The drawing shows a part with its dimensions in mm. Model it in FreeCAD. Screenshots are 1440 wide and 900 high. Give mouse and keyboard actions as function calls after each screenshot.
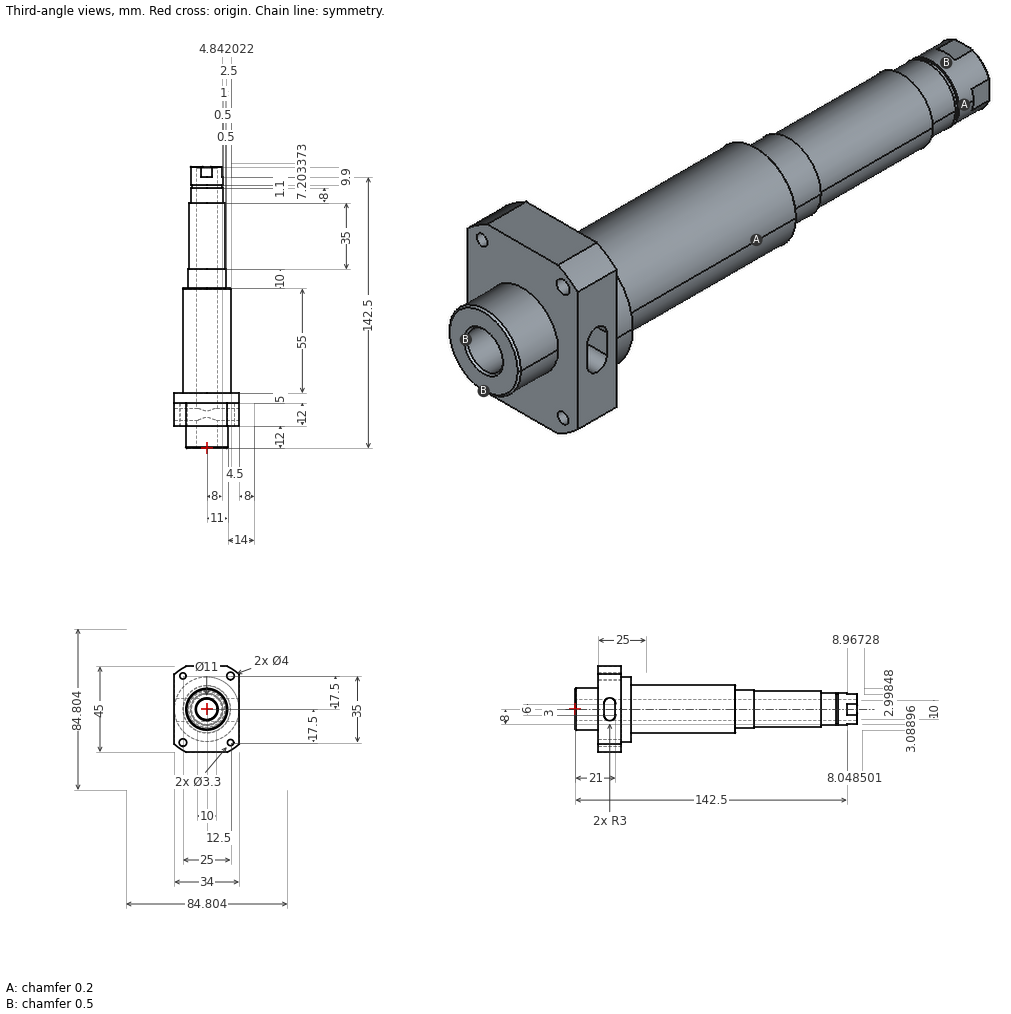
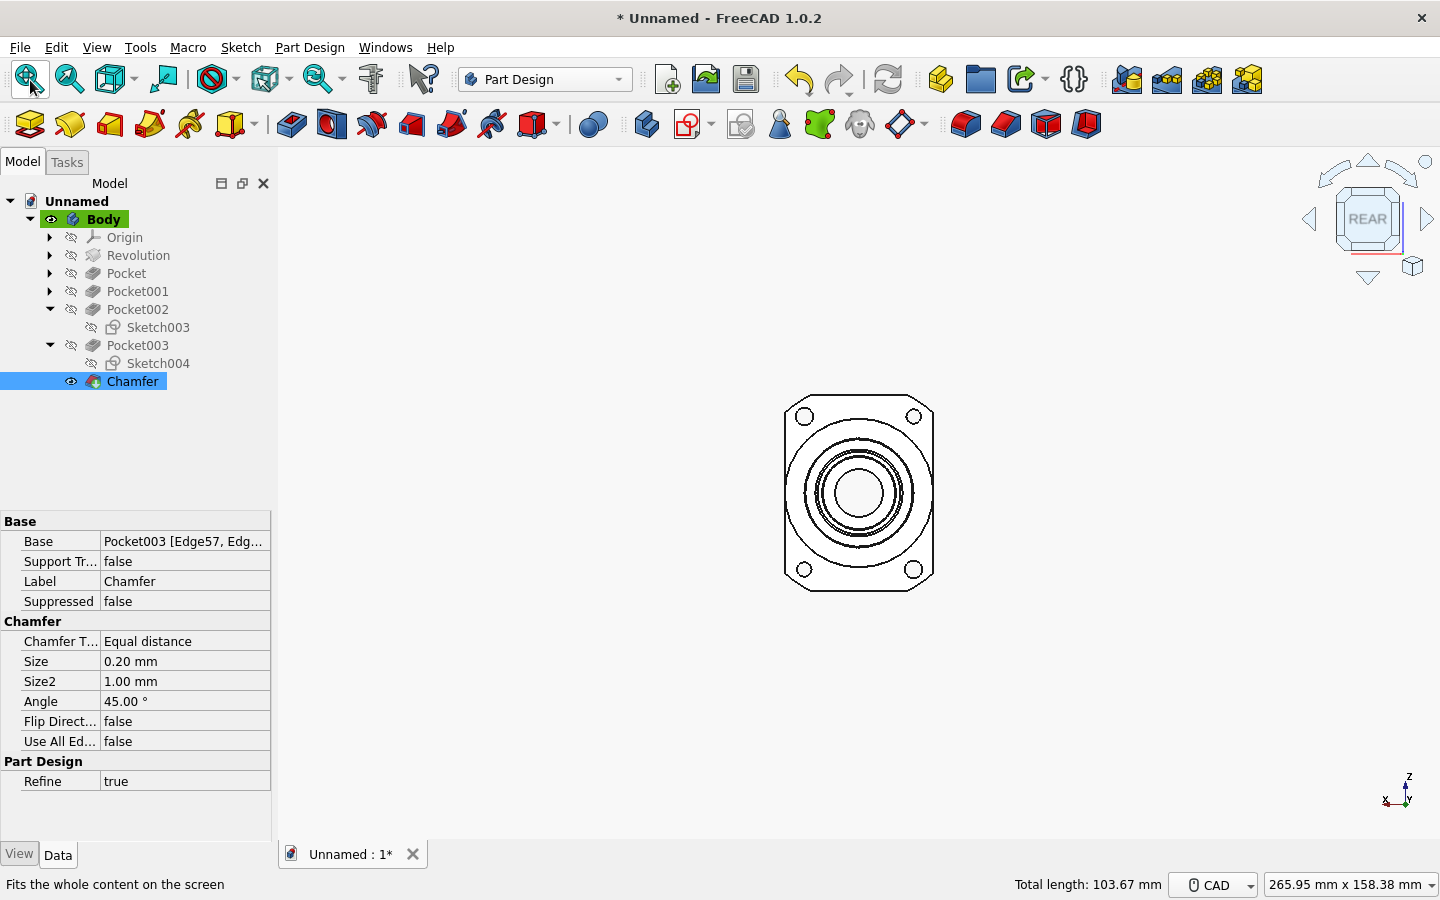
click(883, 492, ctrl)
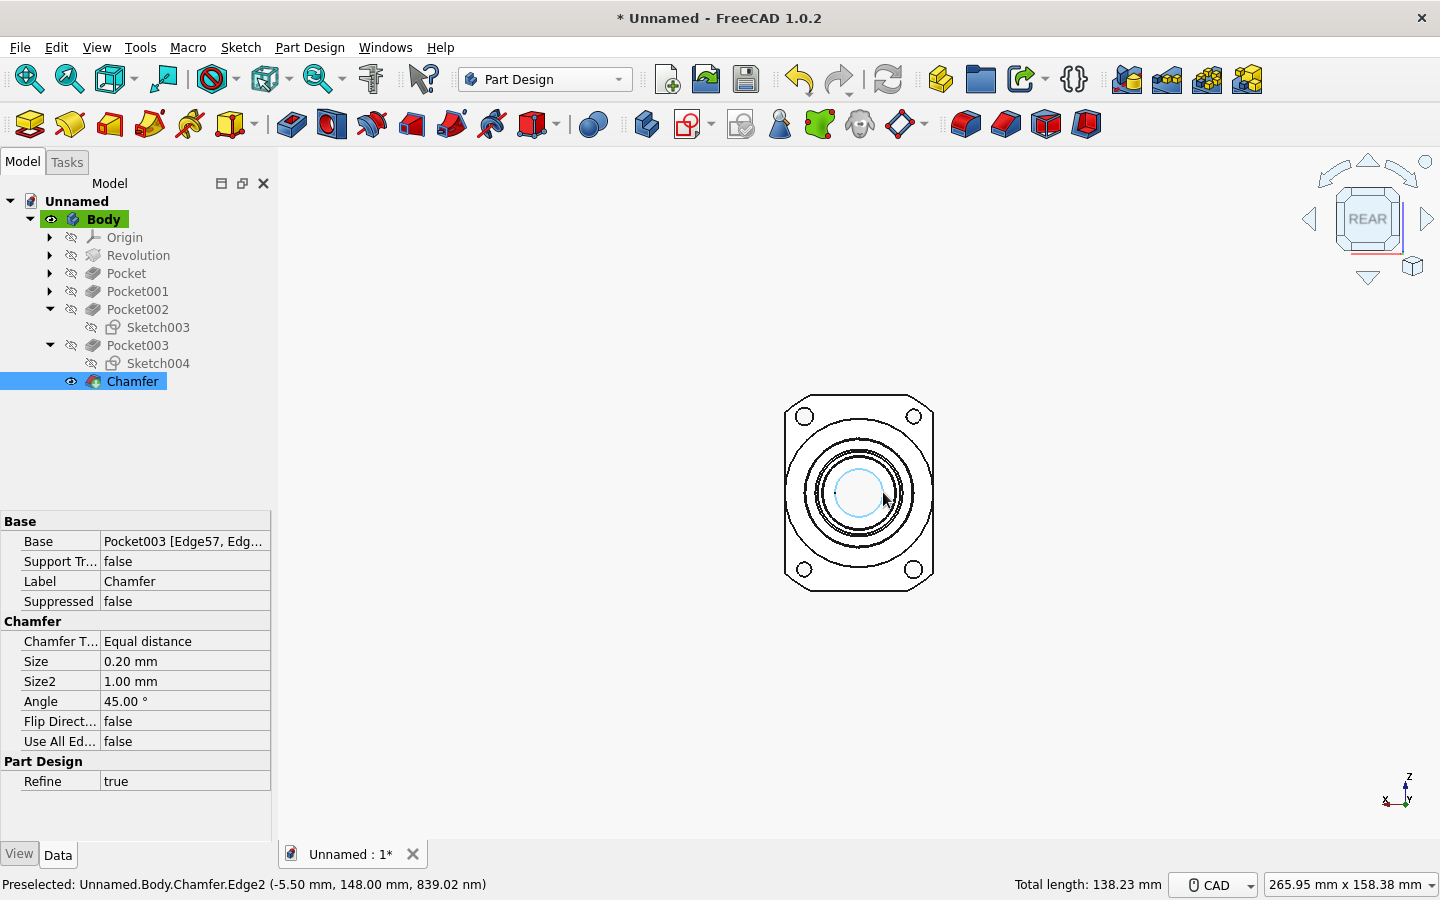
click(1006, 124)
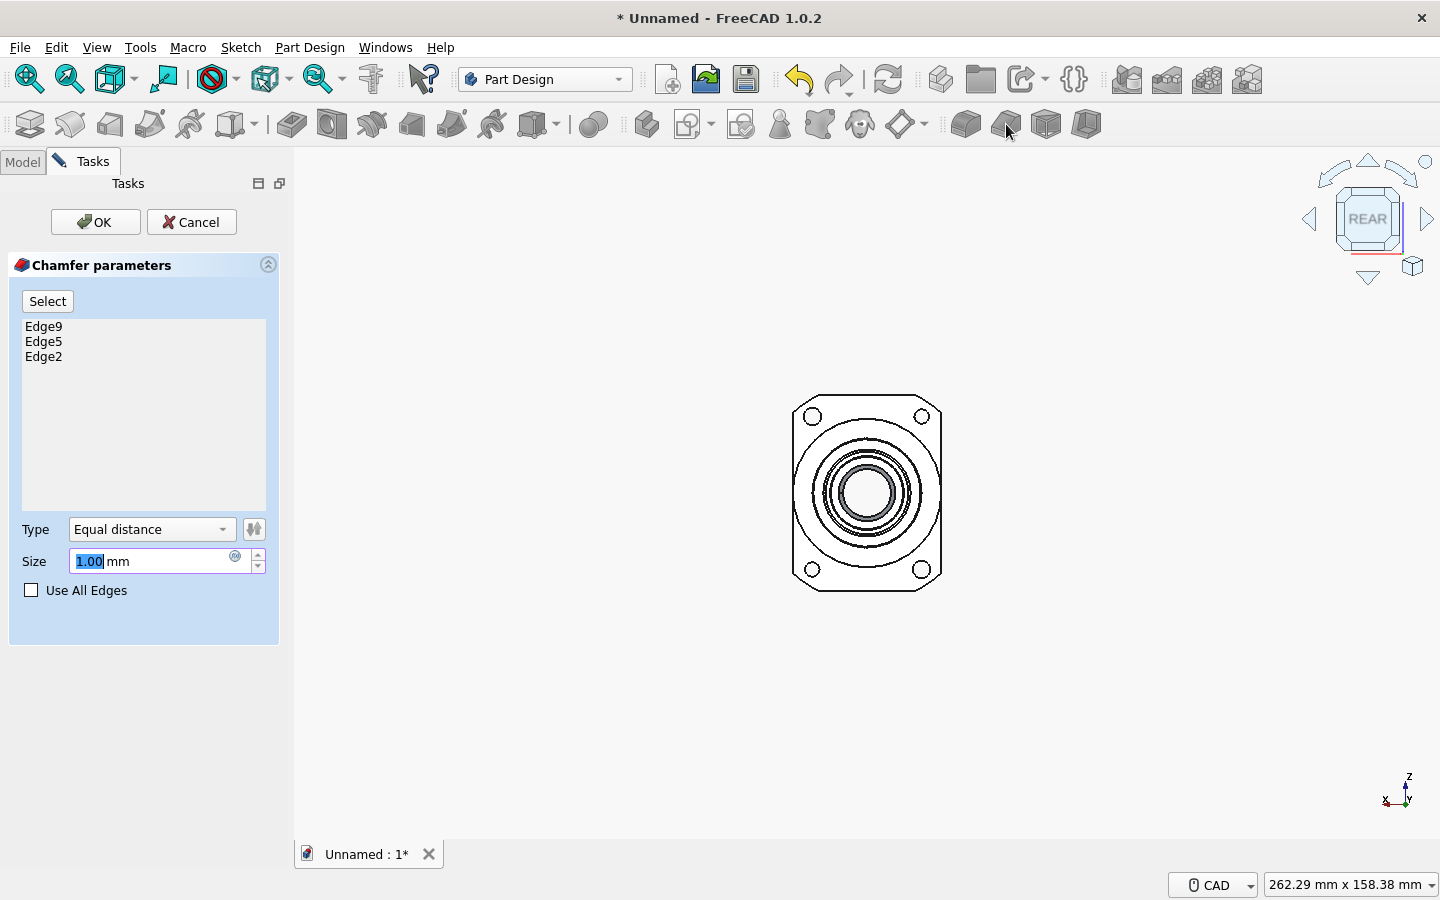
text(0.5)
key(Tab)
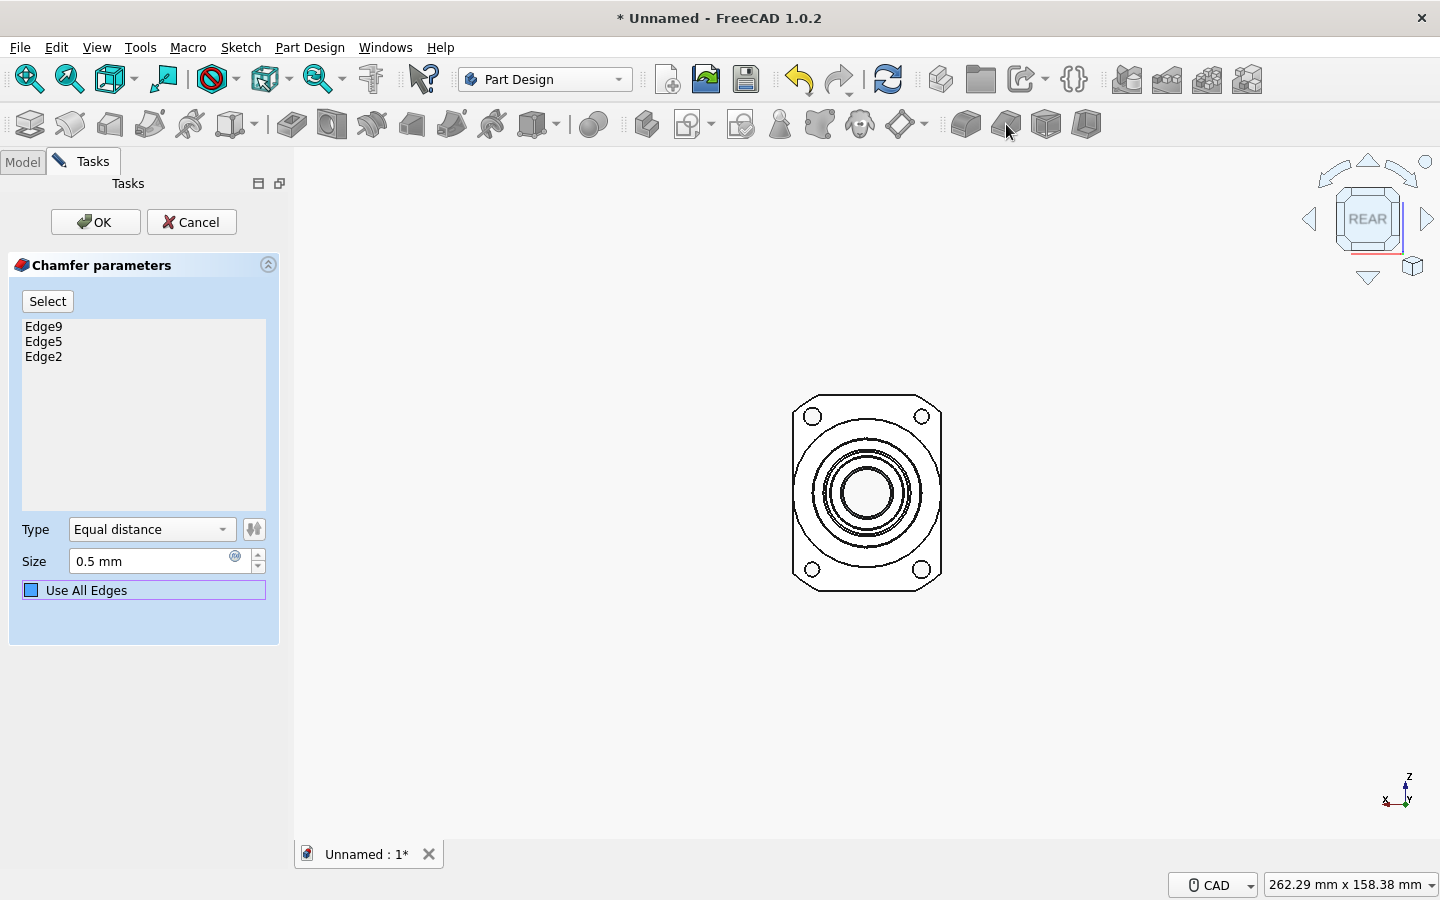
click(96, 222)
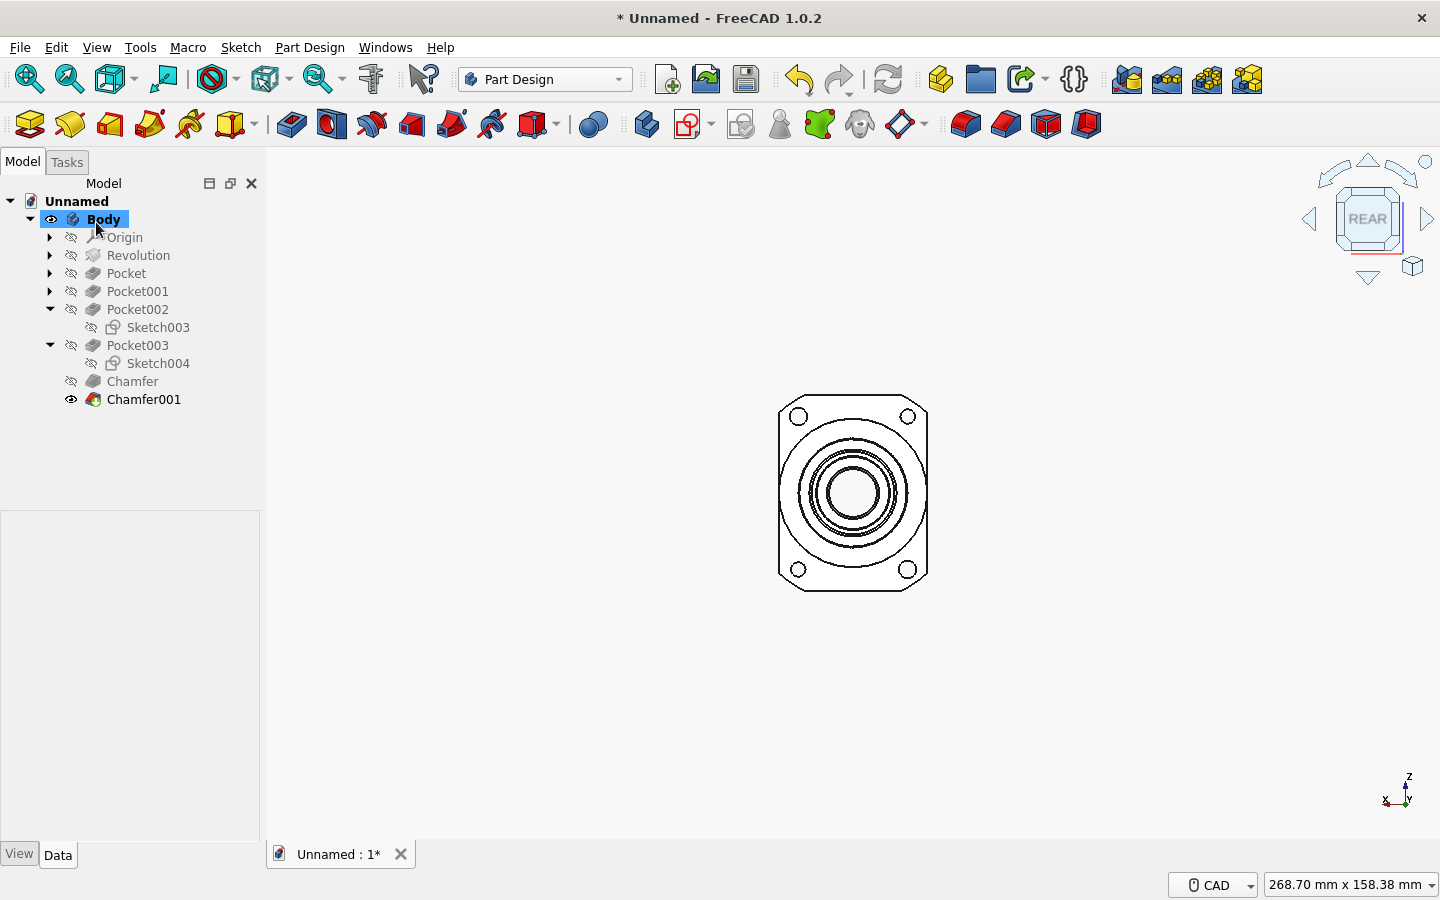
click(30, 80)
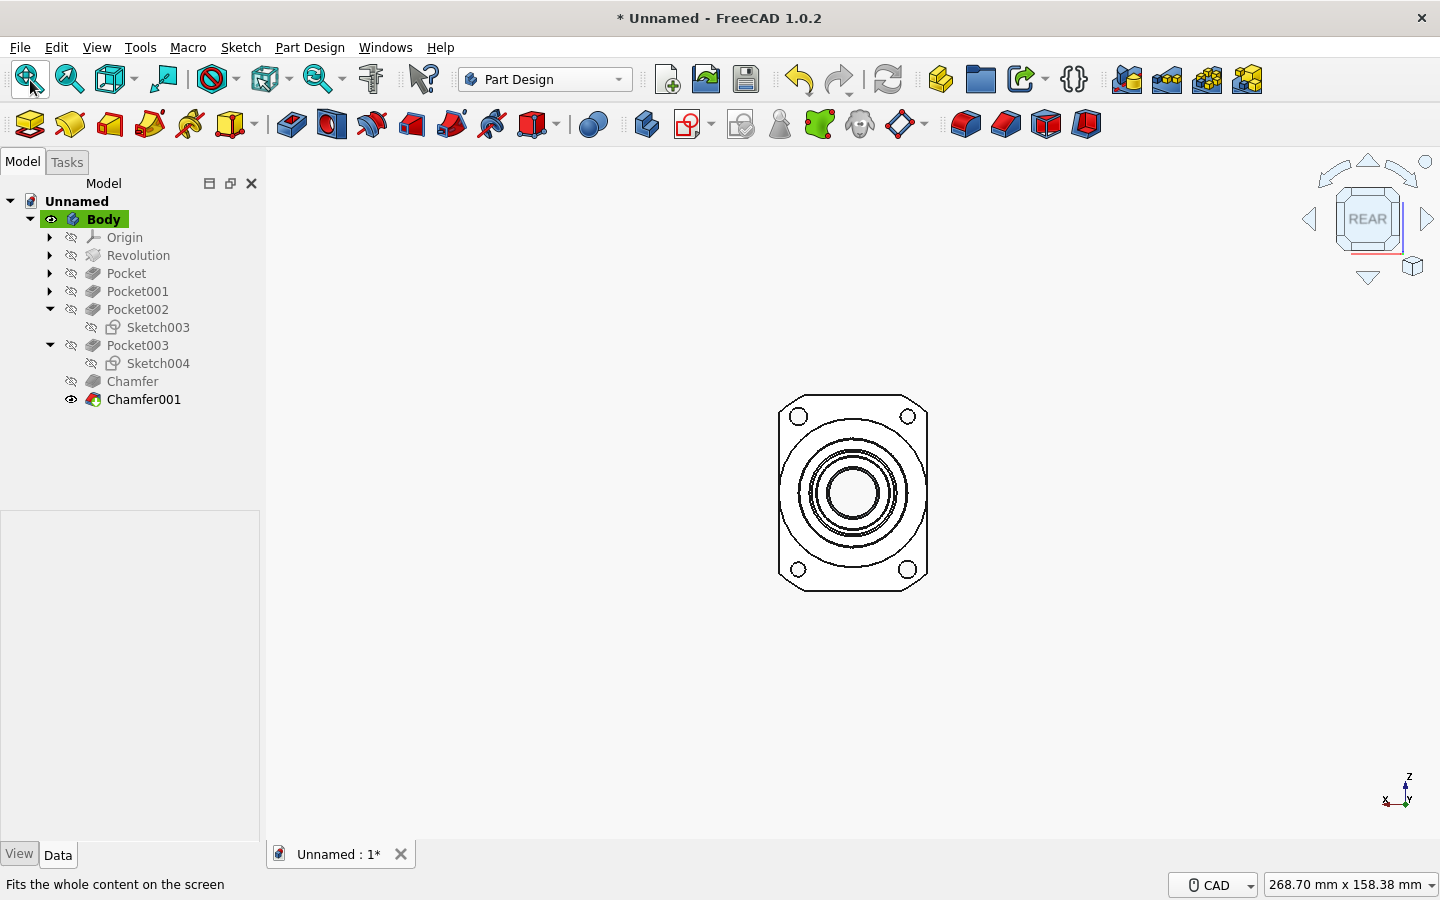
click(688, 124)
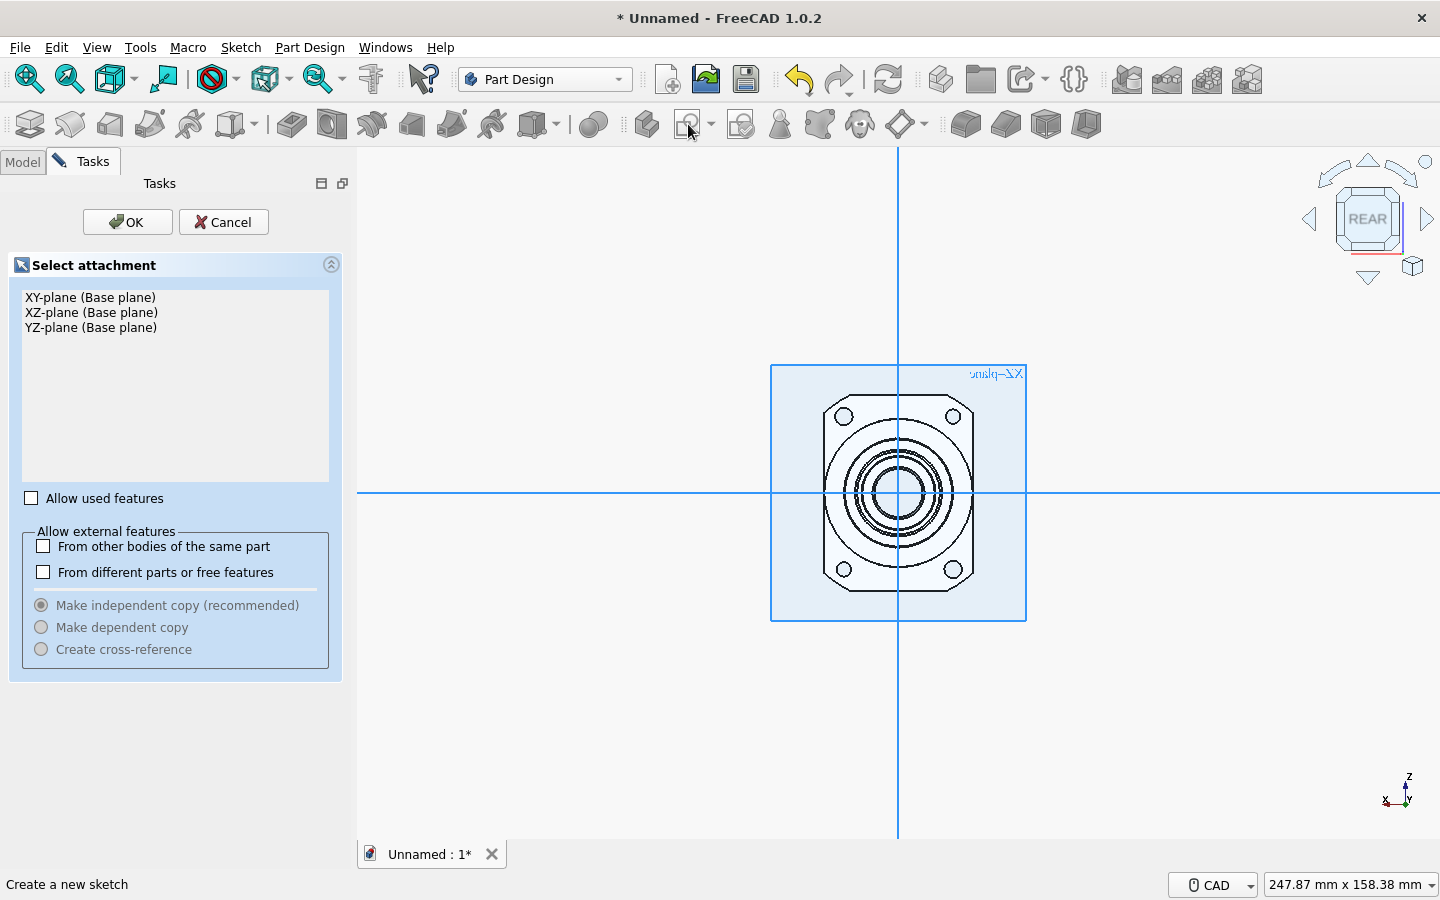
click(82, 298)